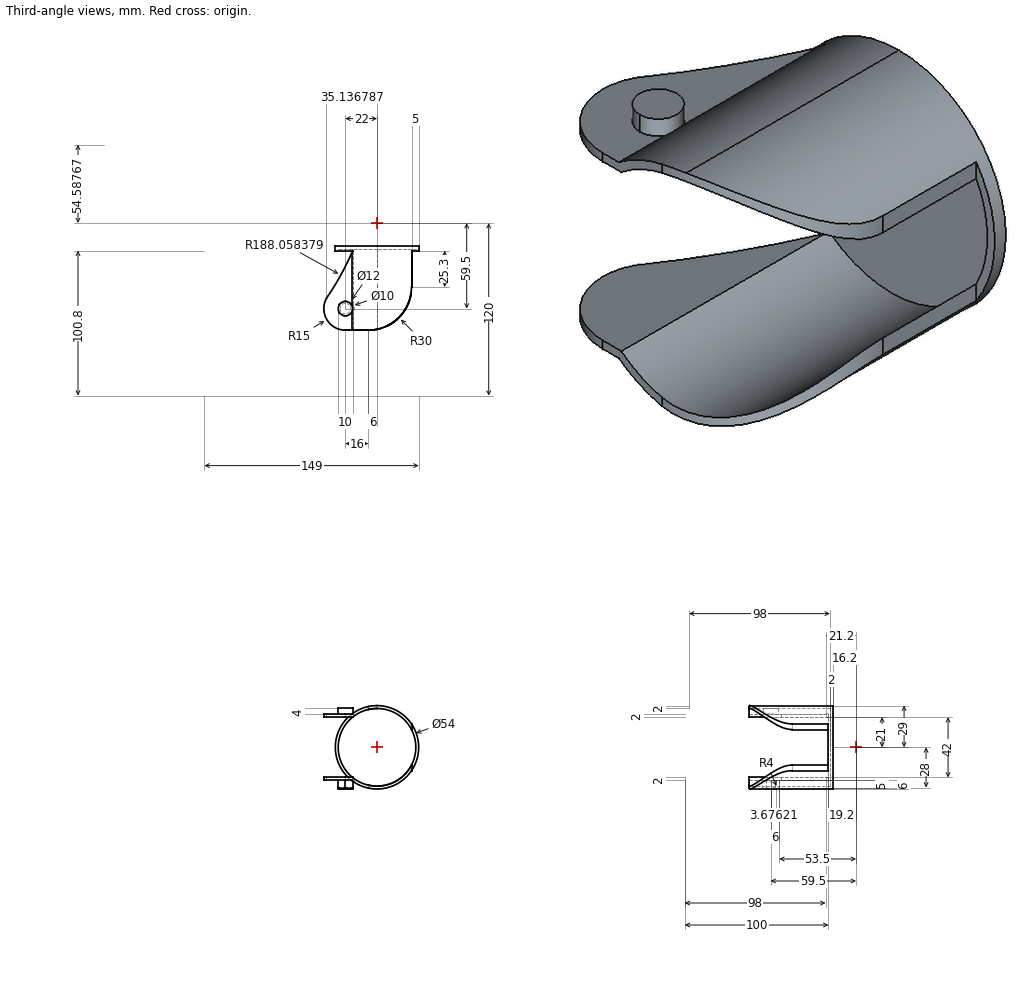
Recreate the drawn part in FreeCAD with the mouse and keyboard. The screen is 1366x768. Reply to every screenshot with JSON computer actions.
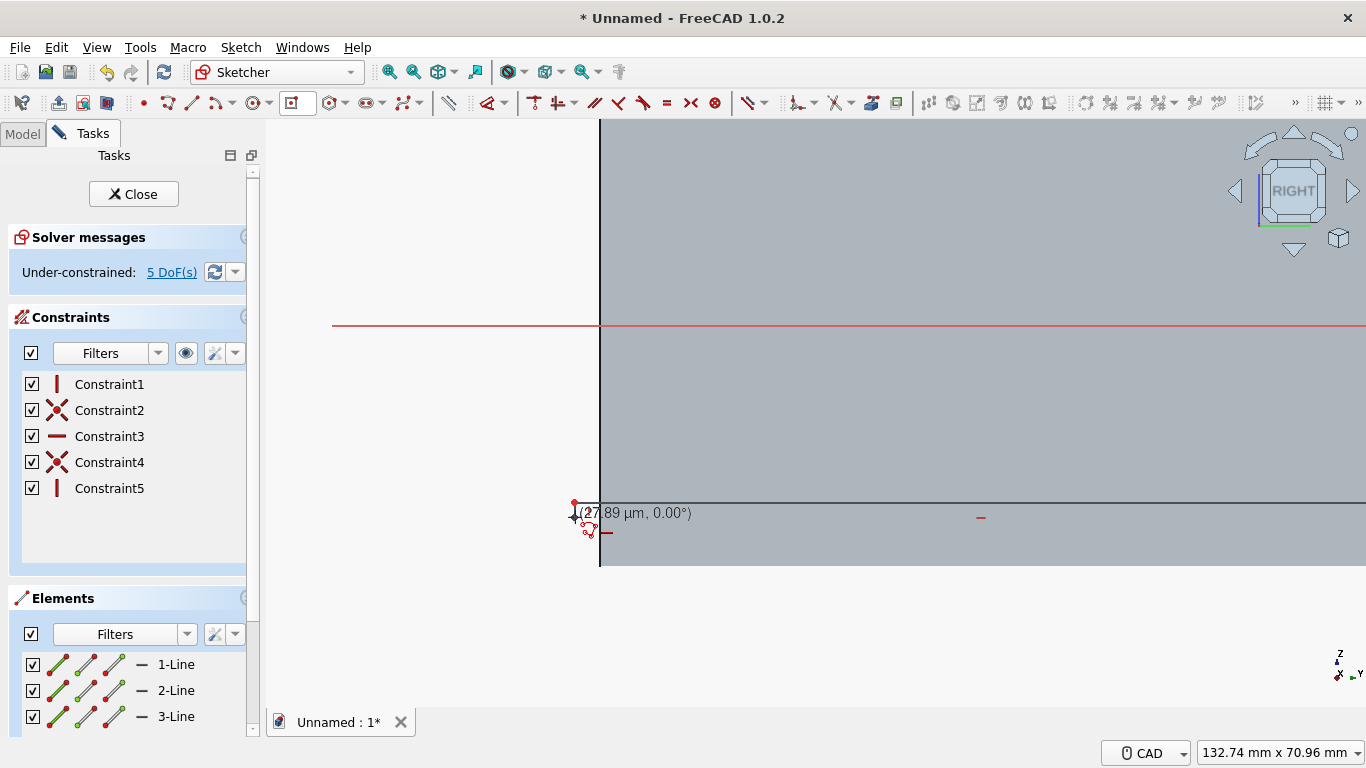
{"action": "scroll", "coordinate": [294, 589], "scroll_direction": "down", "scroll_amount": 2}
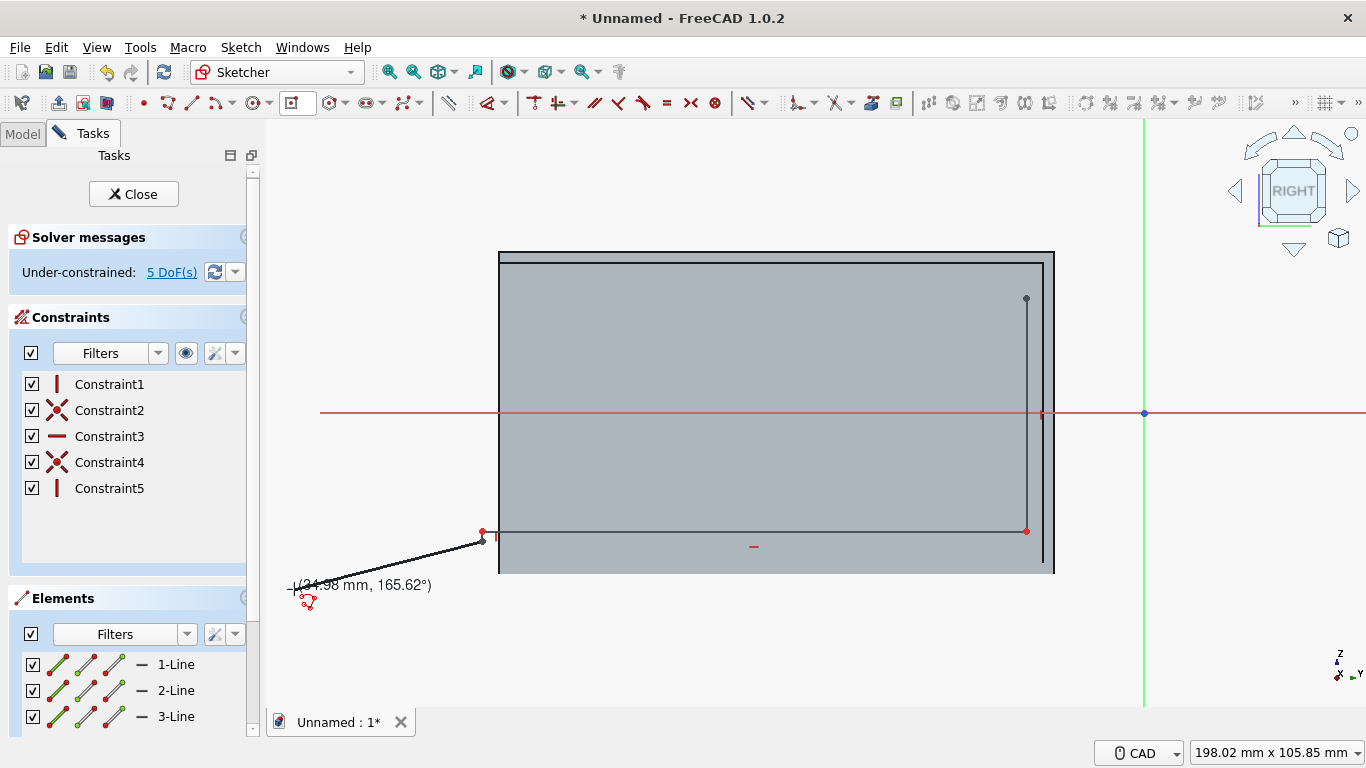
{"action": "left_click", "coordinate": [1038, 541]}
{"action": "left_click", "coordinate": [1038, 285]}
{"action": "left_click", "coordinate": [482, 285]}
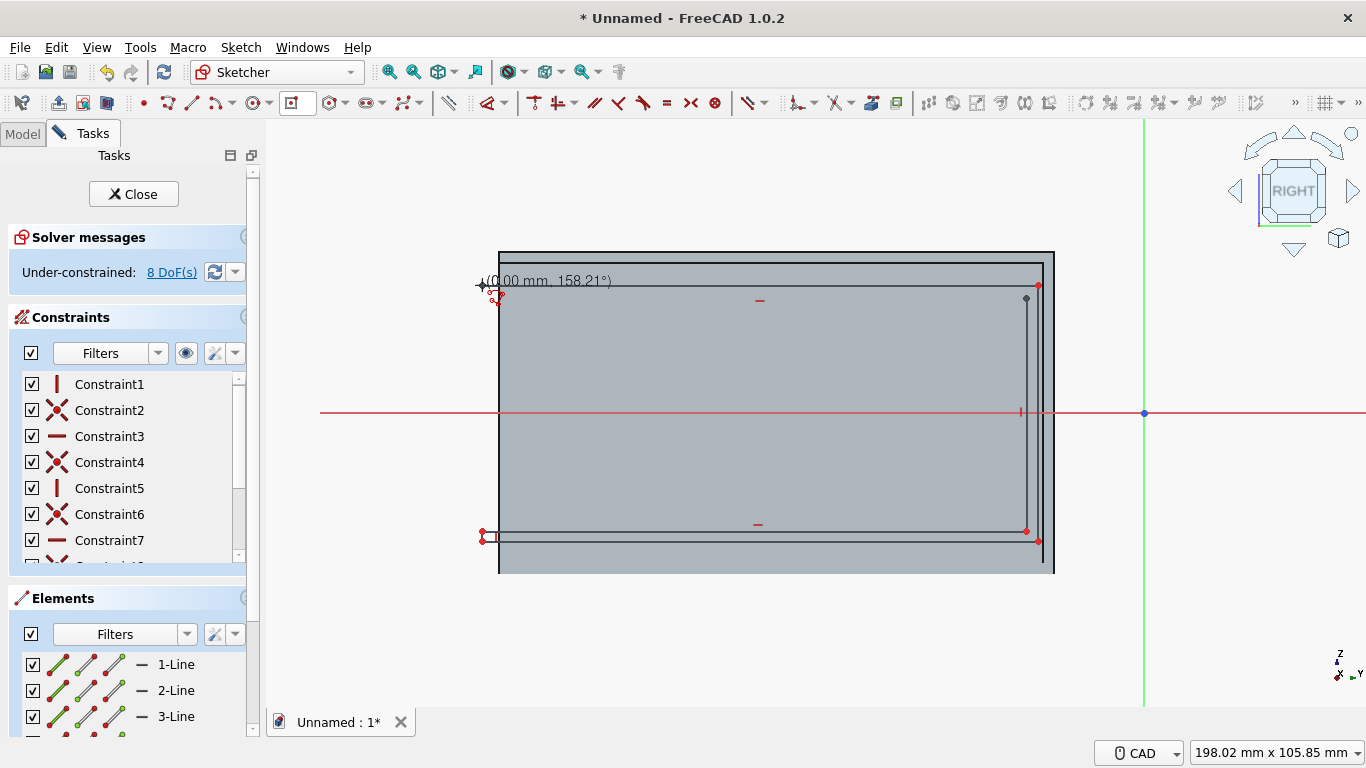
{"action": "scroll", "coordinate": [482, 297], "scroll_direction": "up", "scroll_amount": 2}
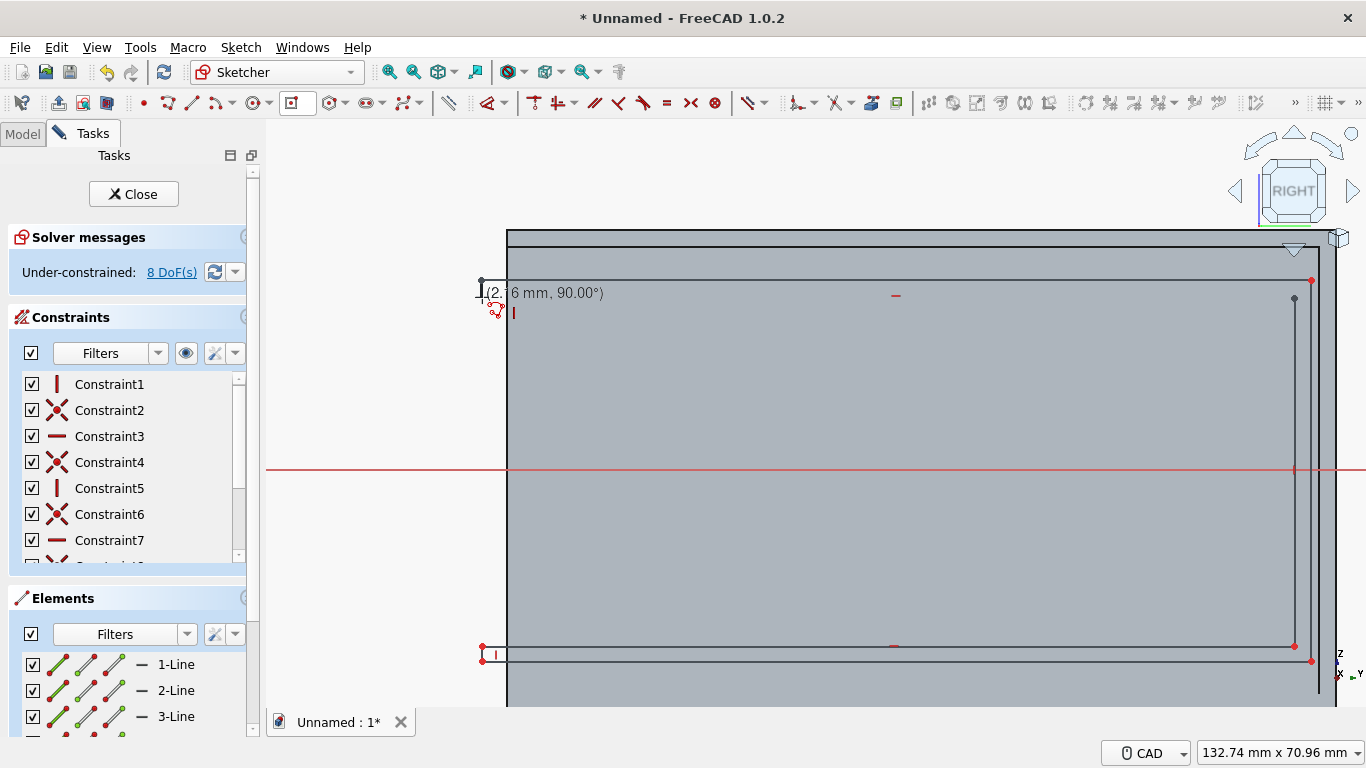
{"action": "left_click", "coordinate": [482, 296]}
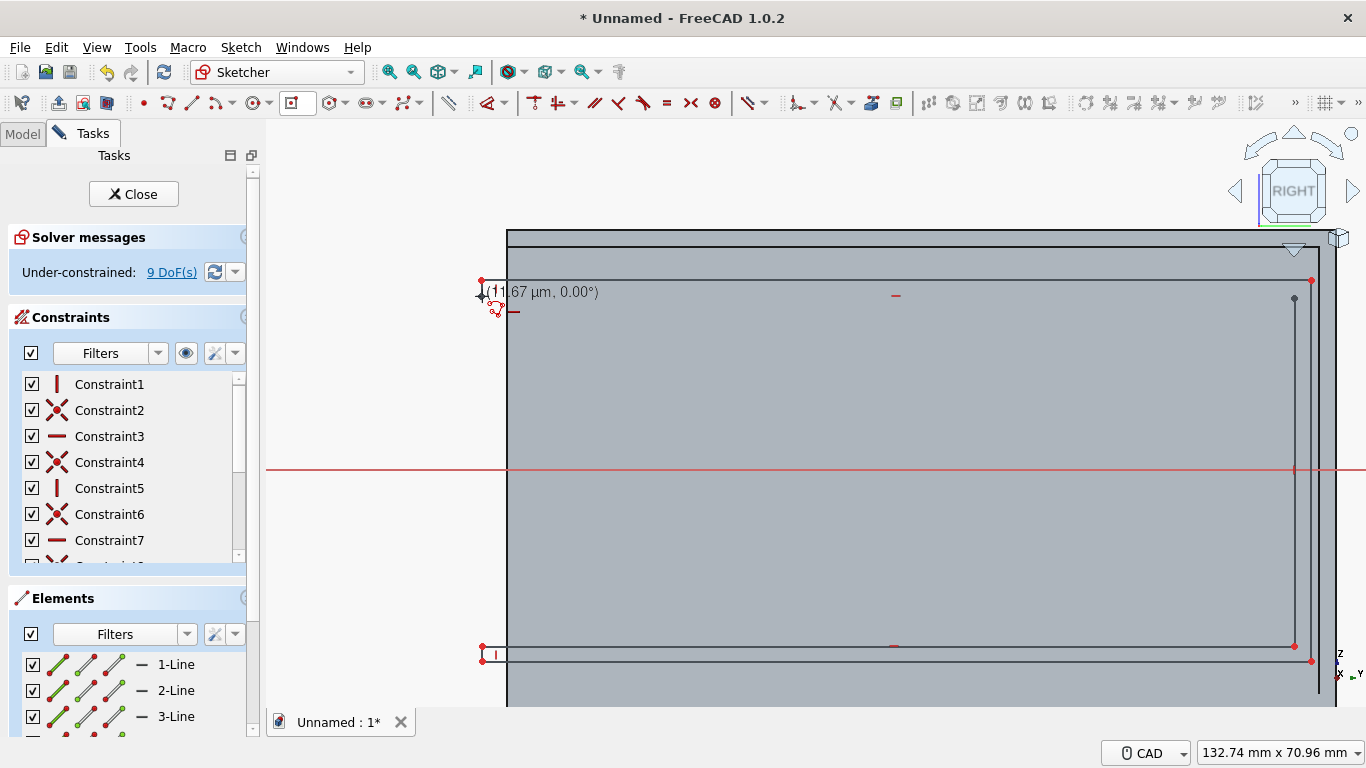
{"action": "scroll", "coordinate": [294, 297], "scroll_direction": "down", "scroll_amount": 2}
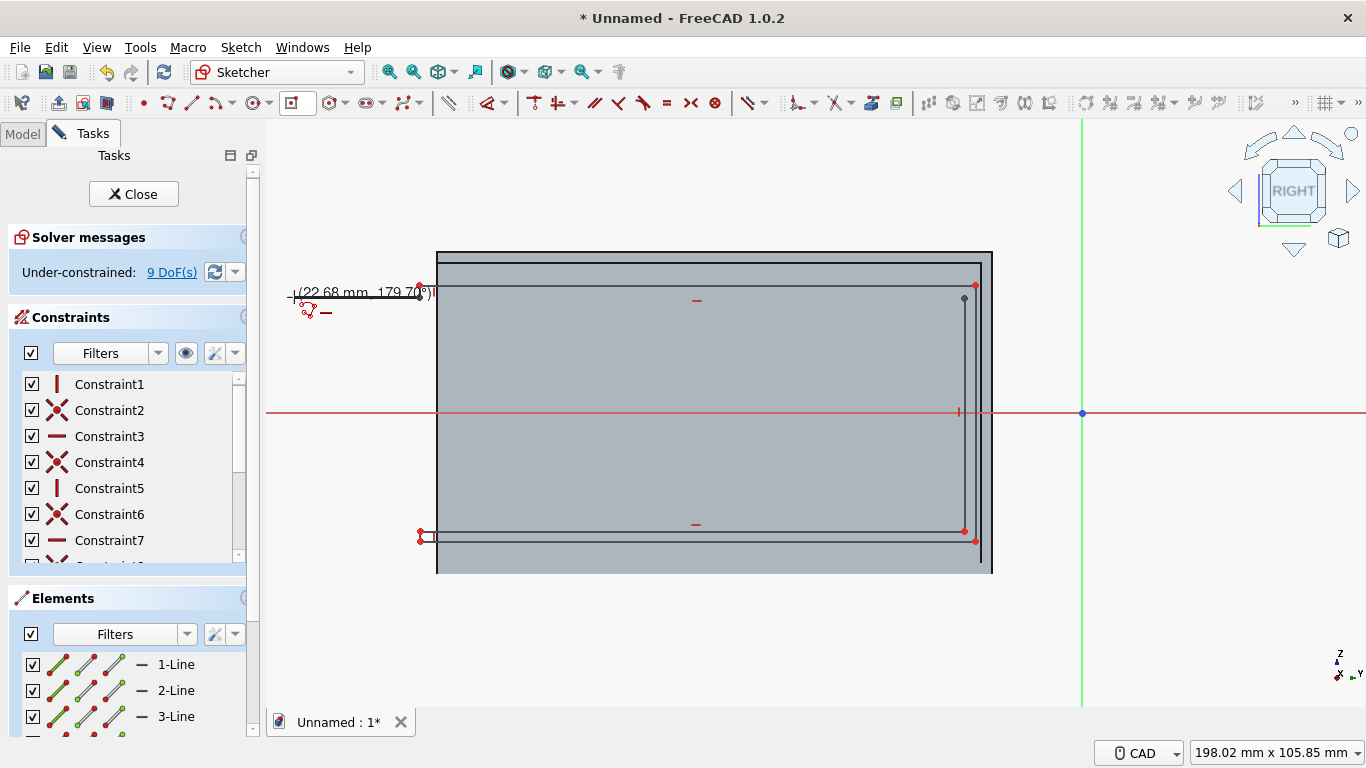
{"action": "scroll", "coordinate": [965, 297], "scroll_direction": "up", "scroll_amount": 2}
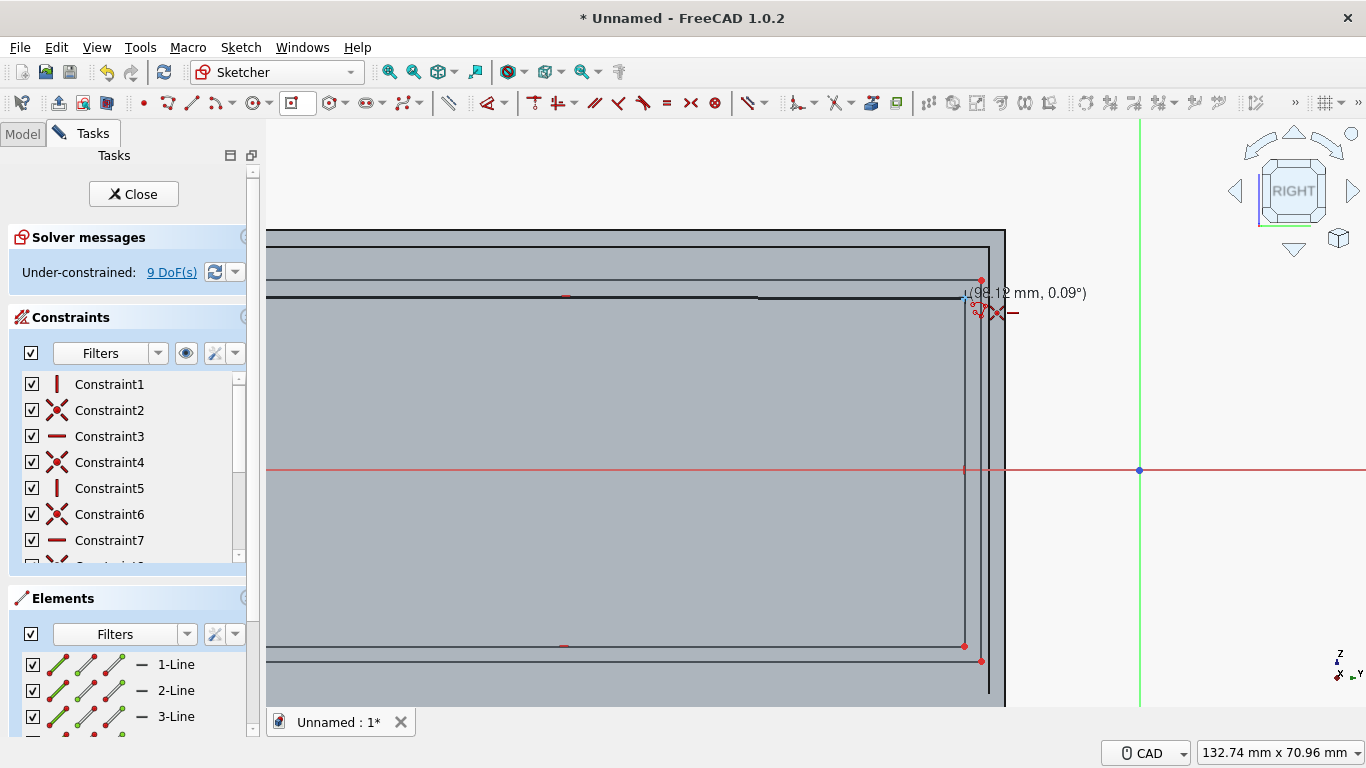
{"action": "left_click", "coordinate": [965, 299]}
{"action": "key", "text": "Escape"}
{"action": "key", "text": "Escape"}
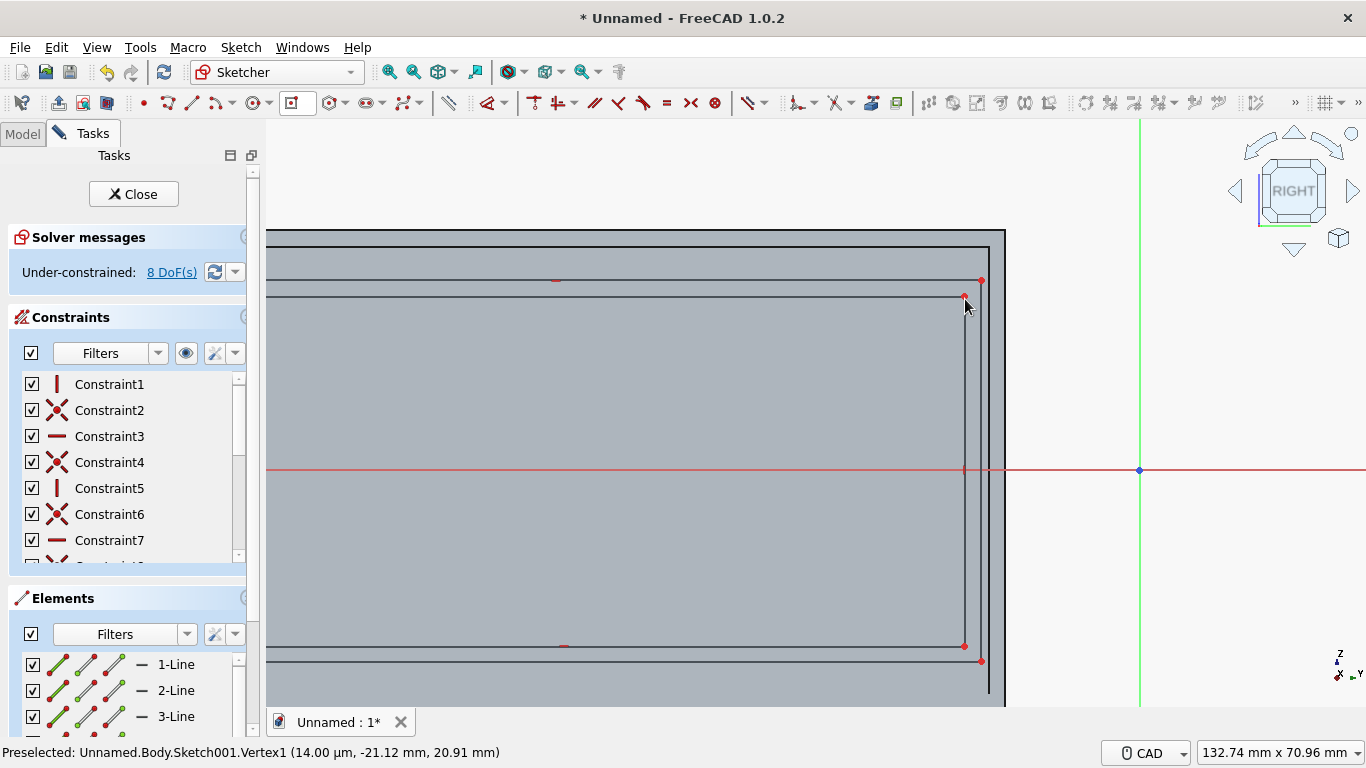
{"action": "left_click", "coordinate": [488, 104]}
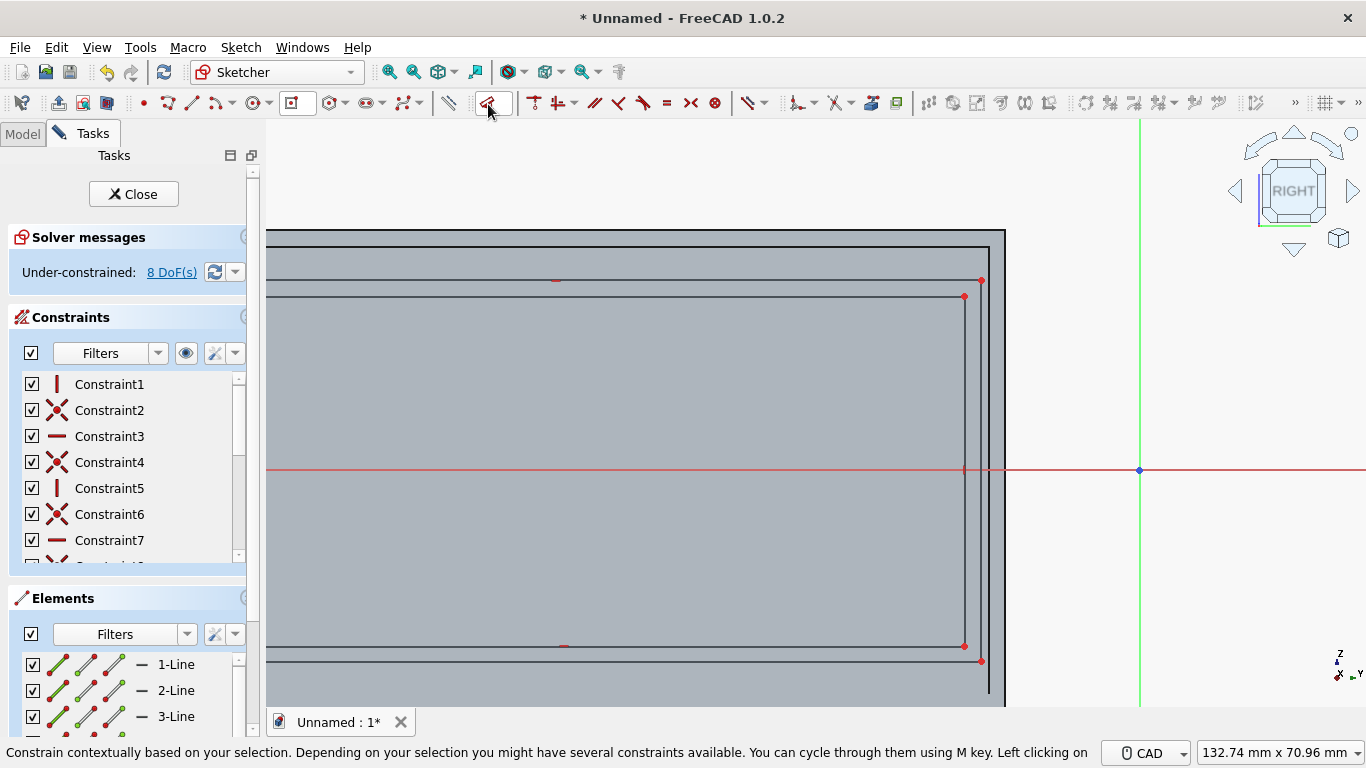
{"action": "scroll", "coordinate": [954, 297], "scroll_direction": "down", "scroll_amount": 2}